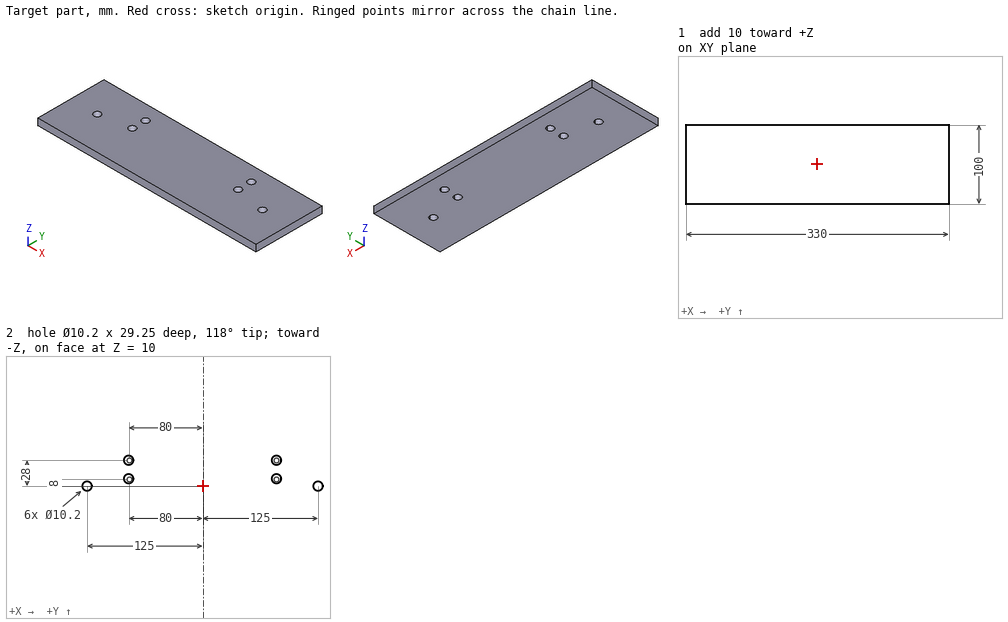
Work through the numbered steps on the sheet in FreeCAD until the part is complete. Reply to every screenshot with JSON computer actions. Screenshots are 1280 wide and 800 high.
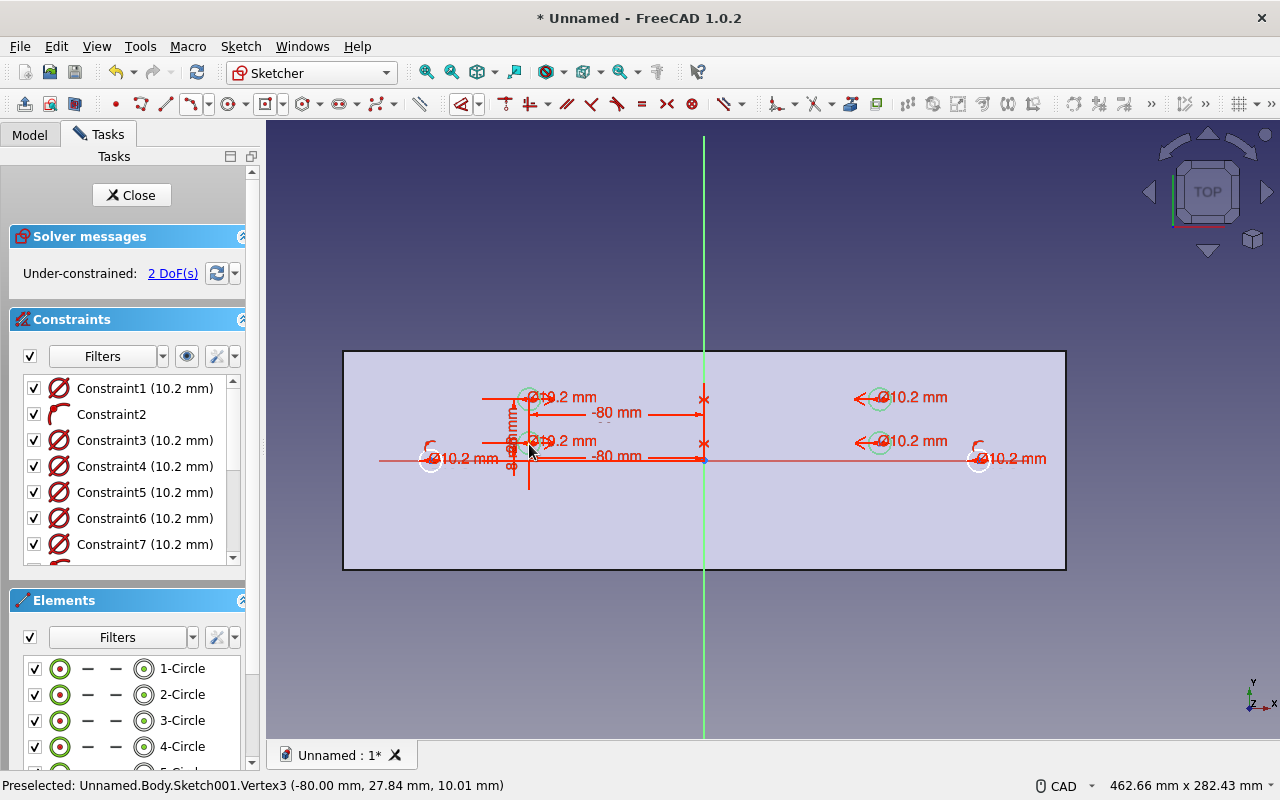
{"action": "left_click", "coordinate": [431, 461]}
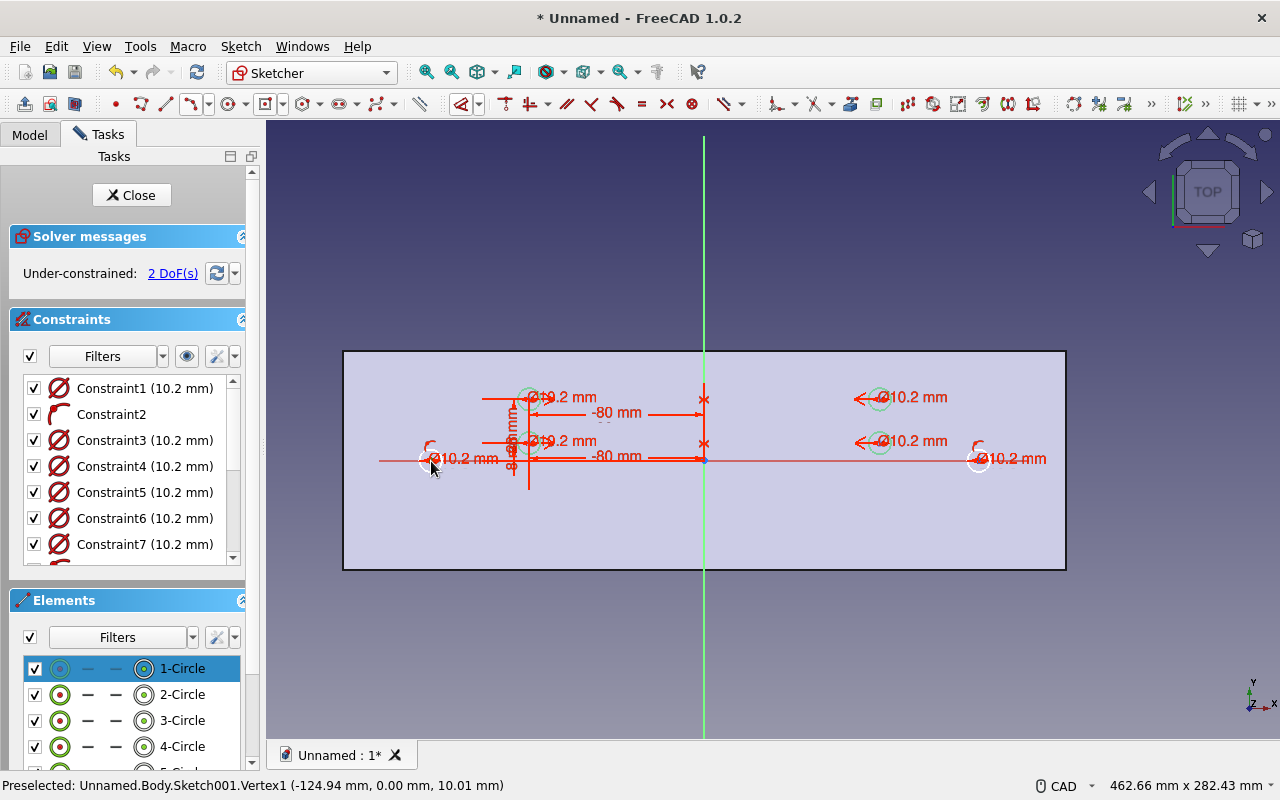
{"action": "left_click", "coordinate": [478, 104]}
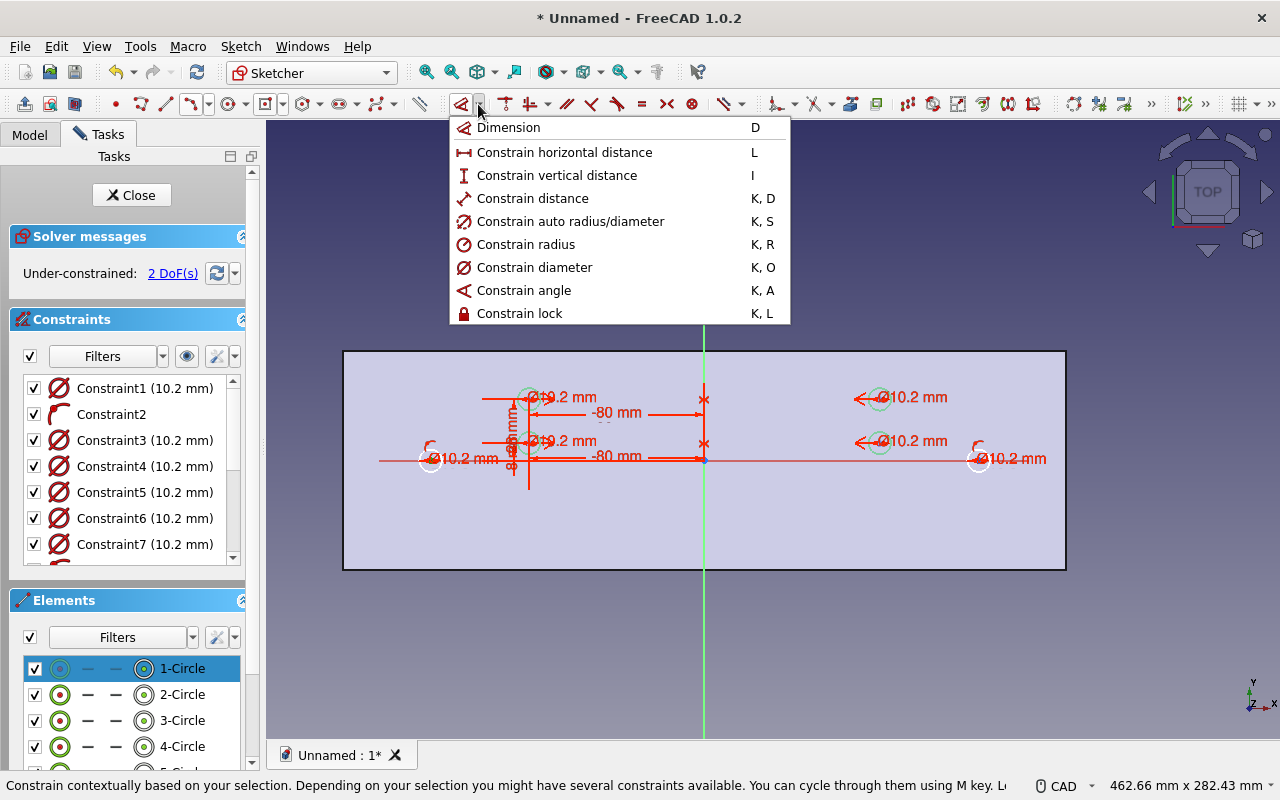
{"action": "left_click", "coordinate": [620, 152]}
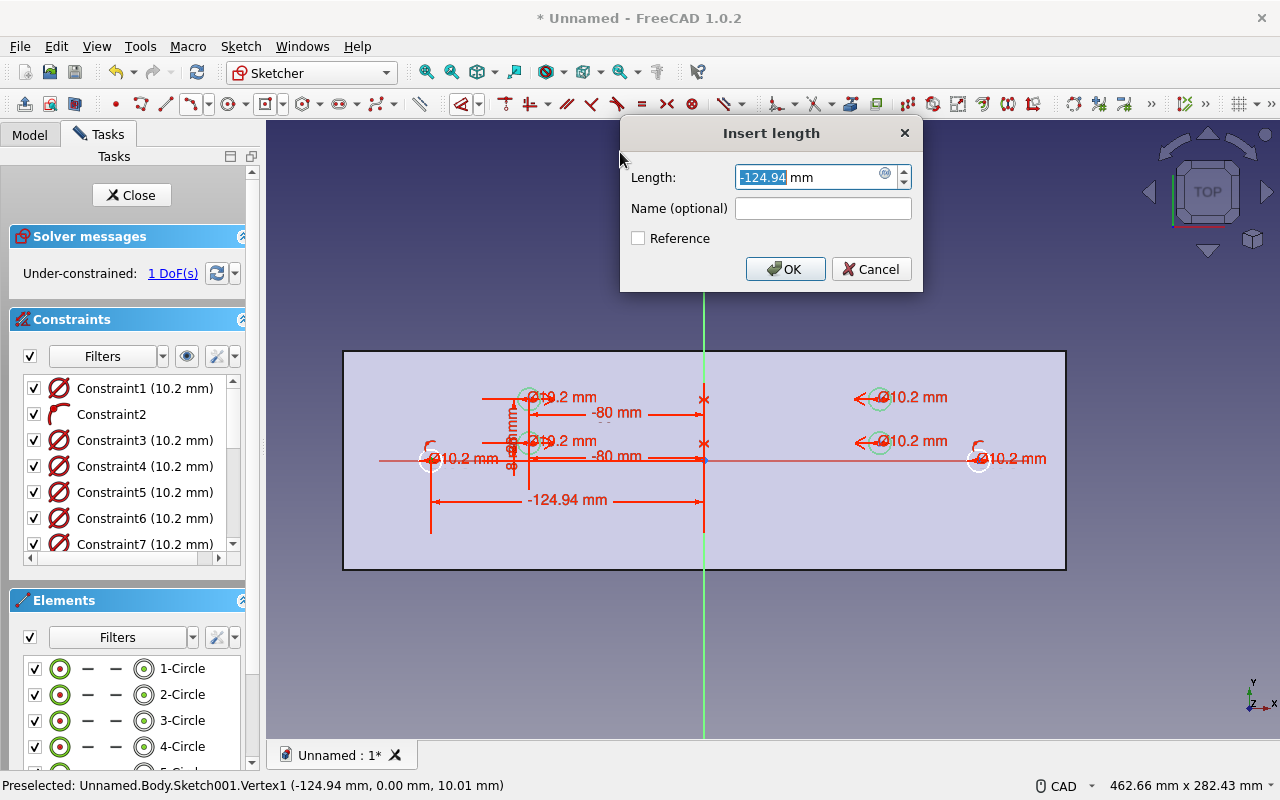
{"action": "type", "text": "-125"}
{"action": "key", "text": "Return"}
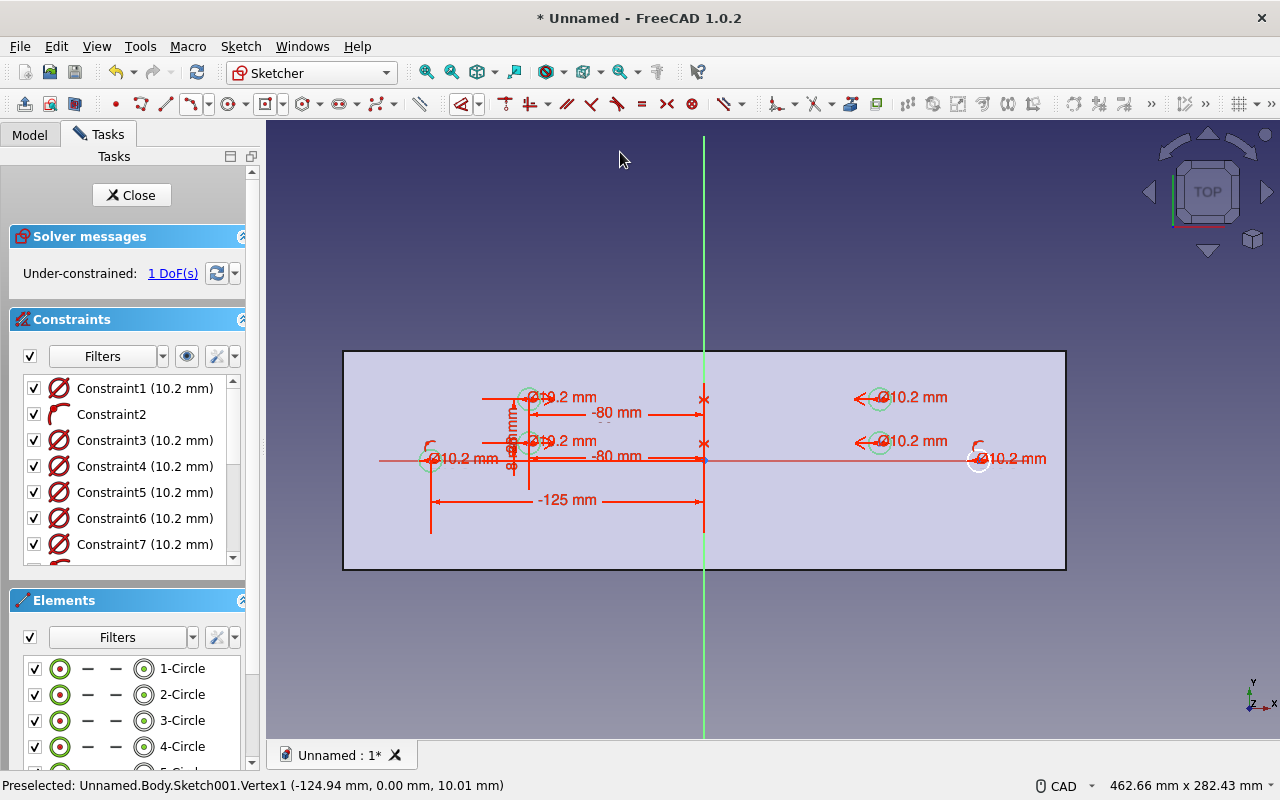
{"action": "left_click", "coordinate": [979, 461]}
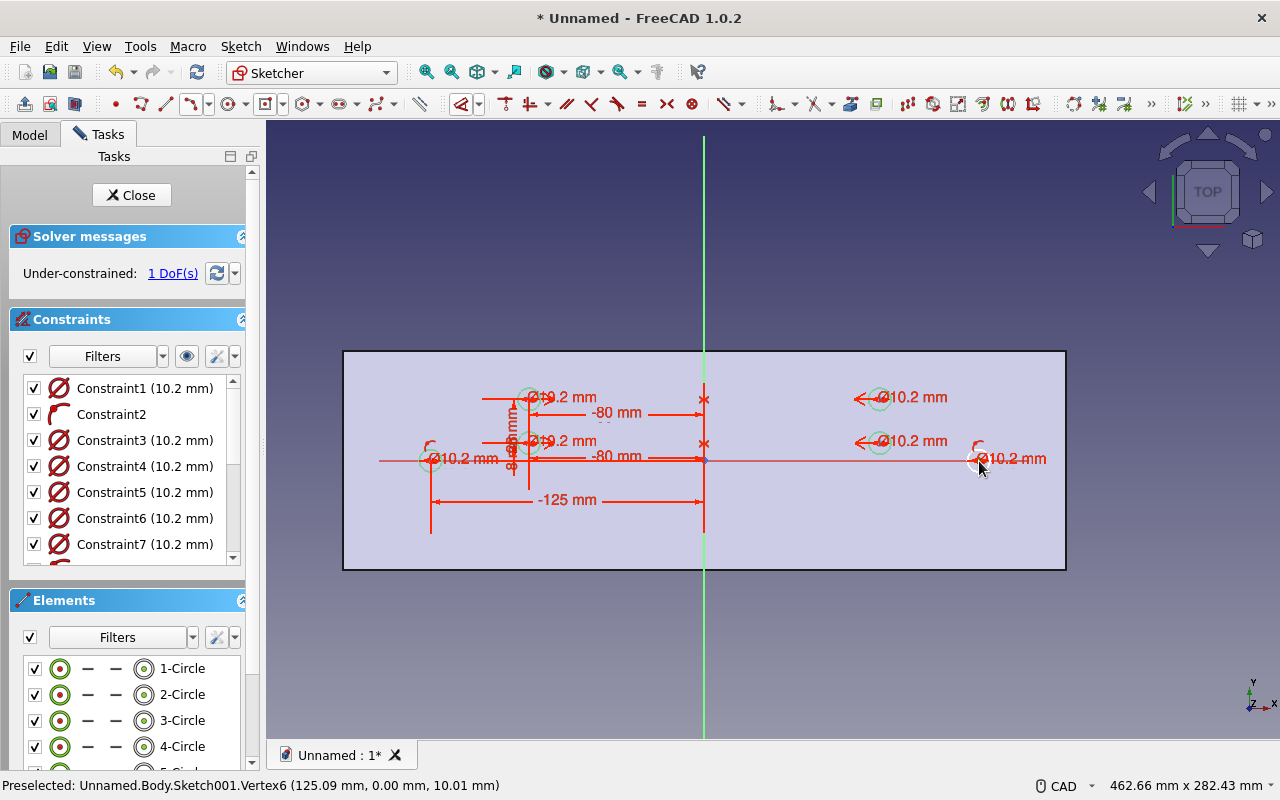
{"action": "left_click", "coordinate": [478, 104]}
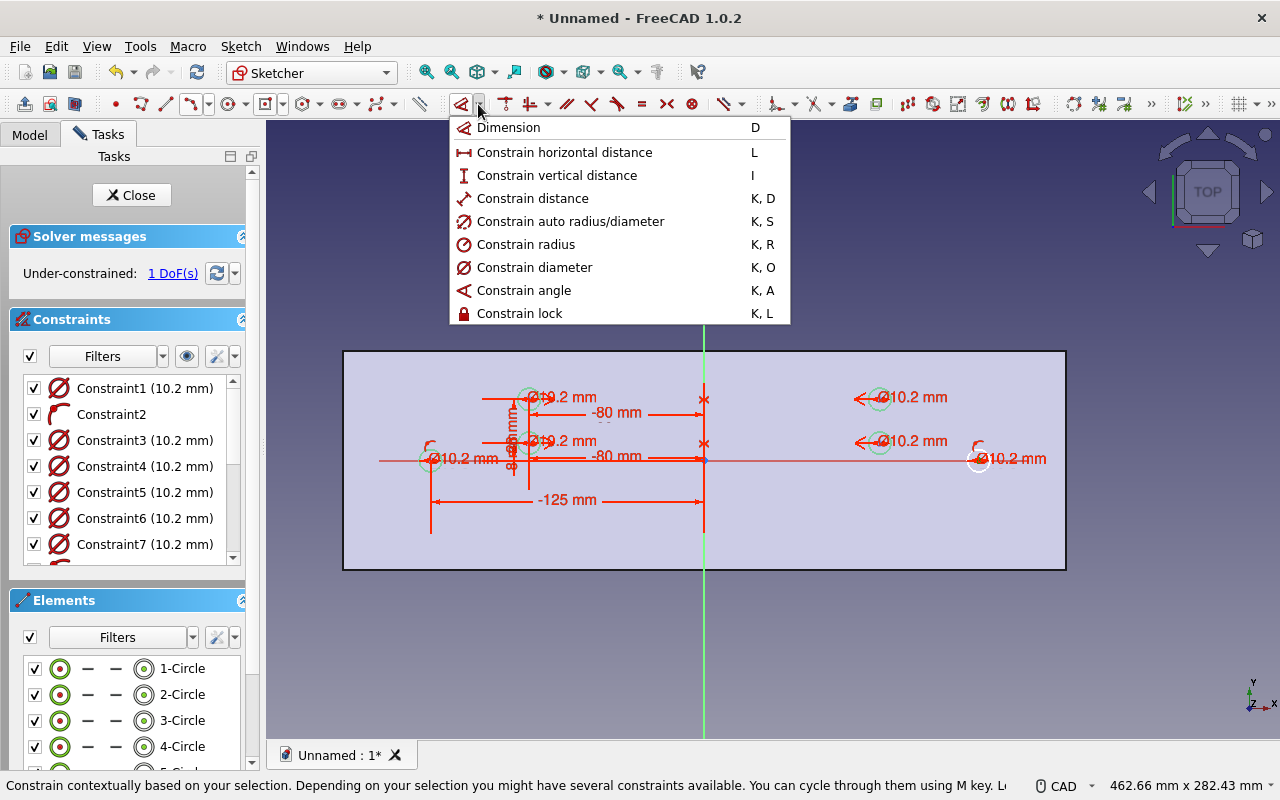
{"action": "left_click", "coordinate": [620, 152]}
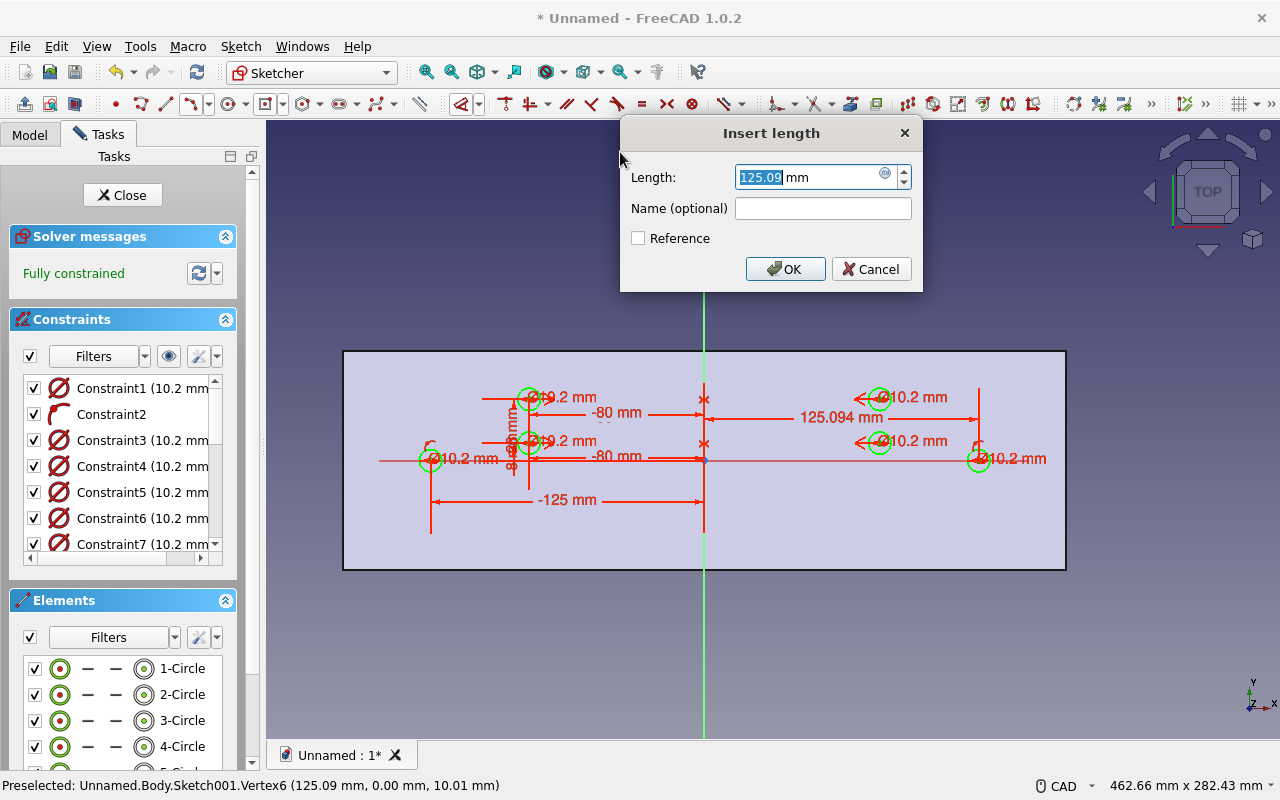
{"action": "type", "text": "125"}
{"action": "key", "text": "Return"}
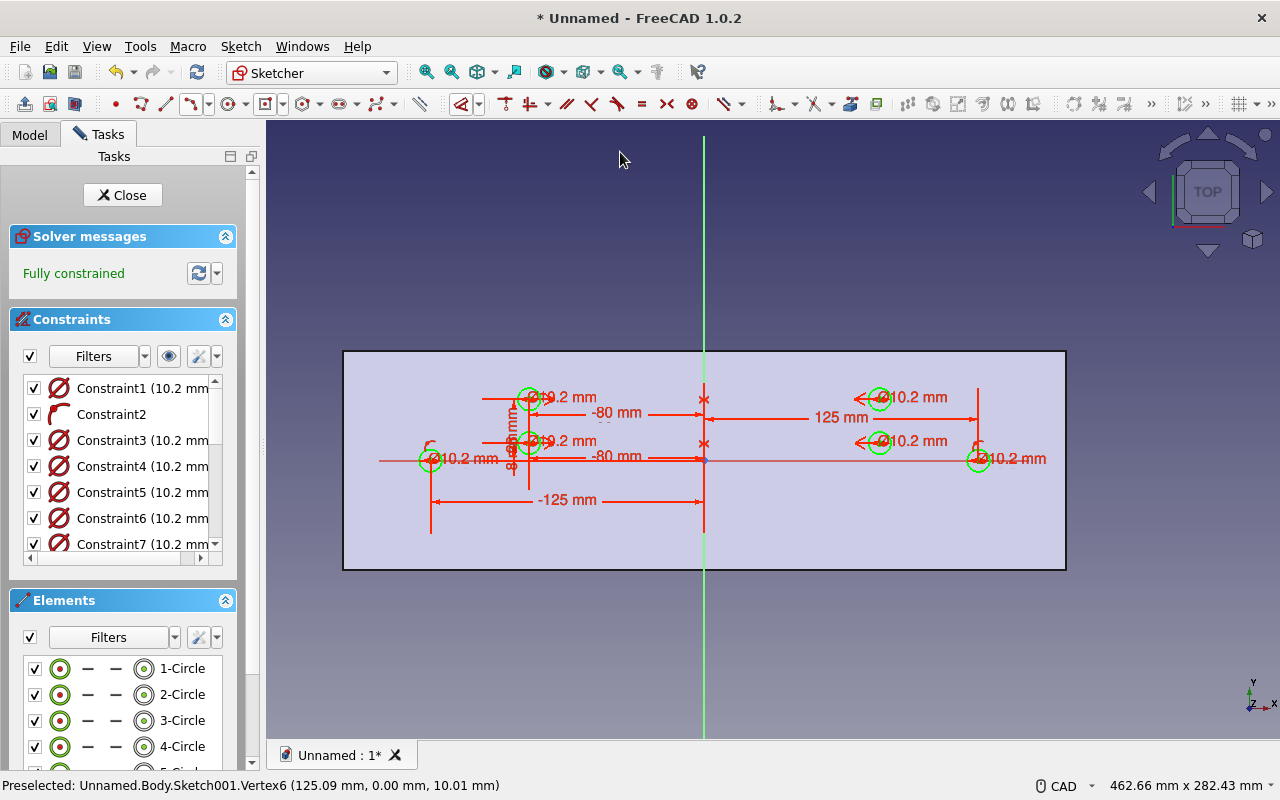
{"action": "left_click", "coordinate": [123, 195]}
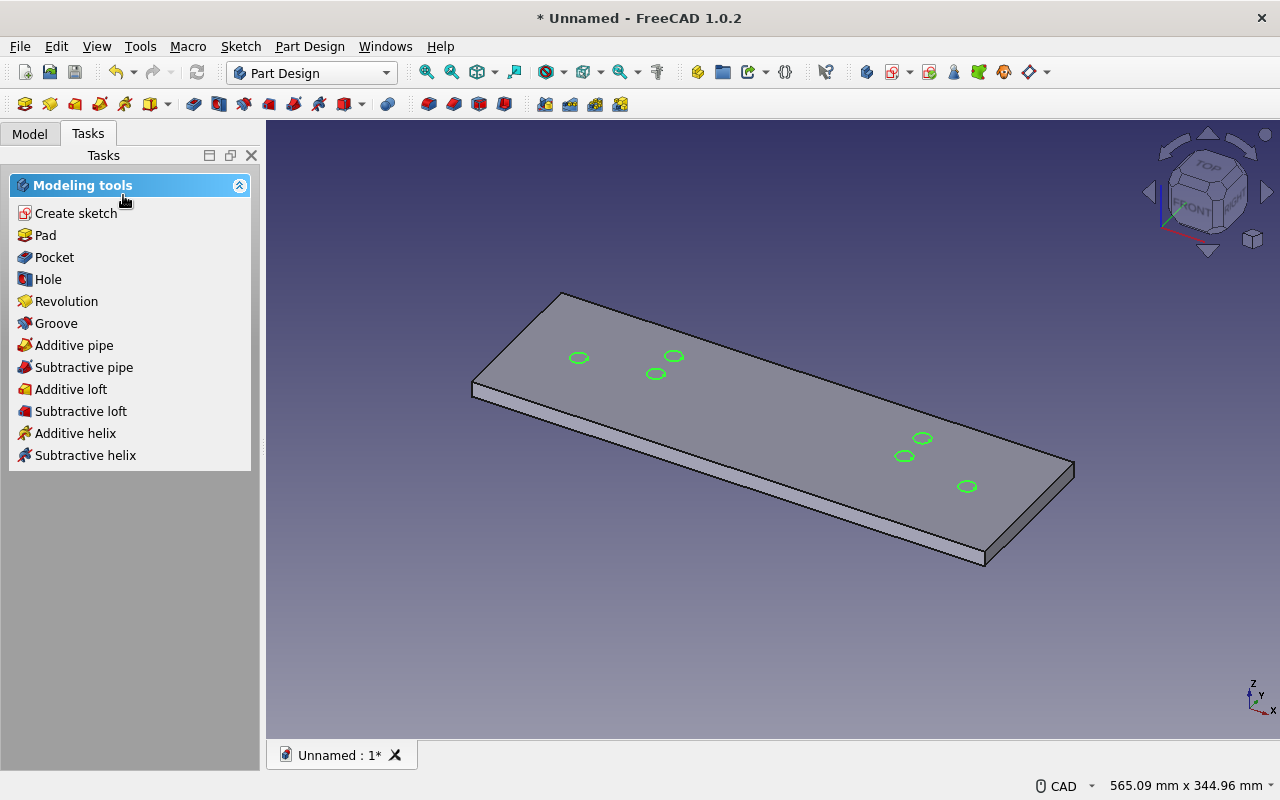
{"action": "left_click", "coordinate": [219, 104]}